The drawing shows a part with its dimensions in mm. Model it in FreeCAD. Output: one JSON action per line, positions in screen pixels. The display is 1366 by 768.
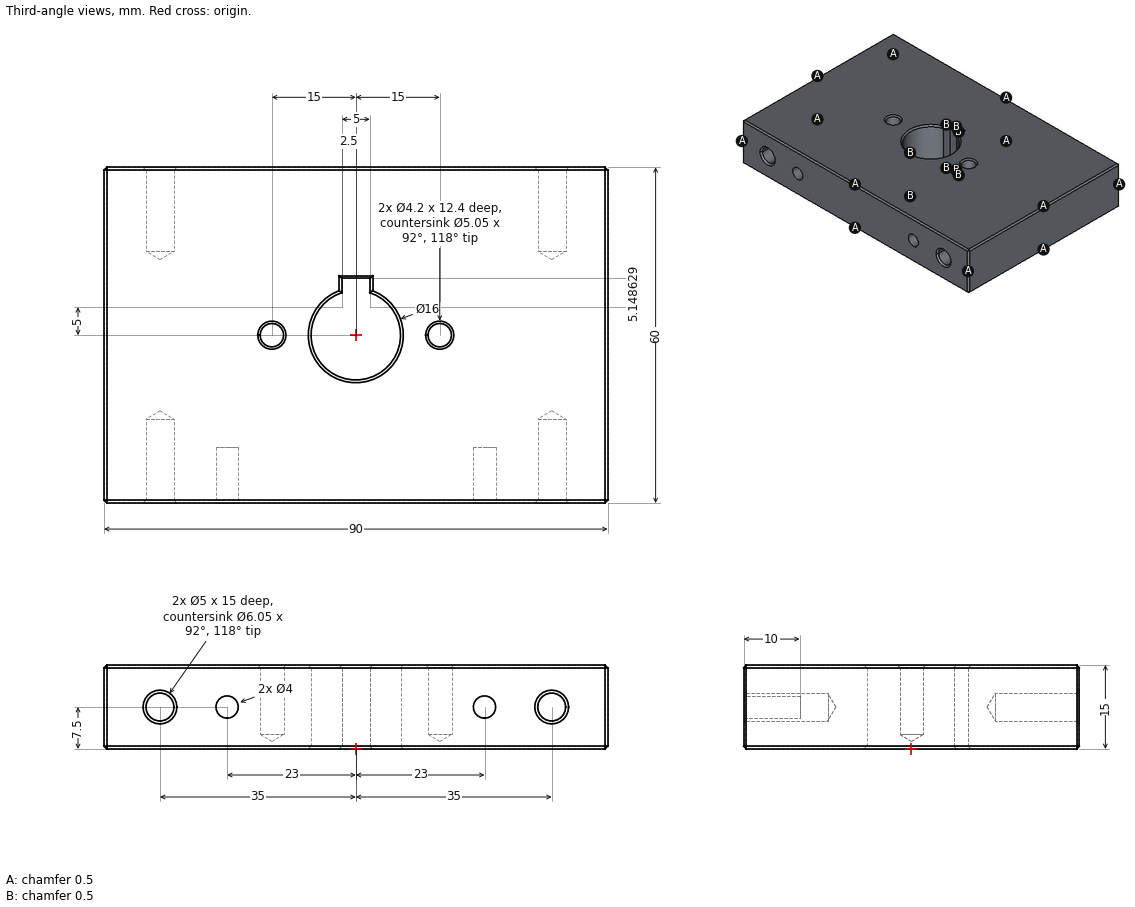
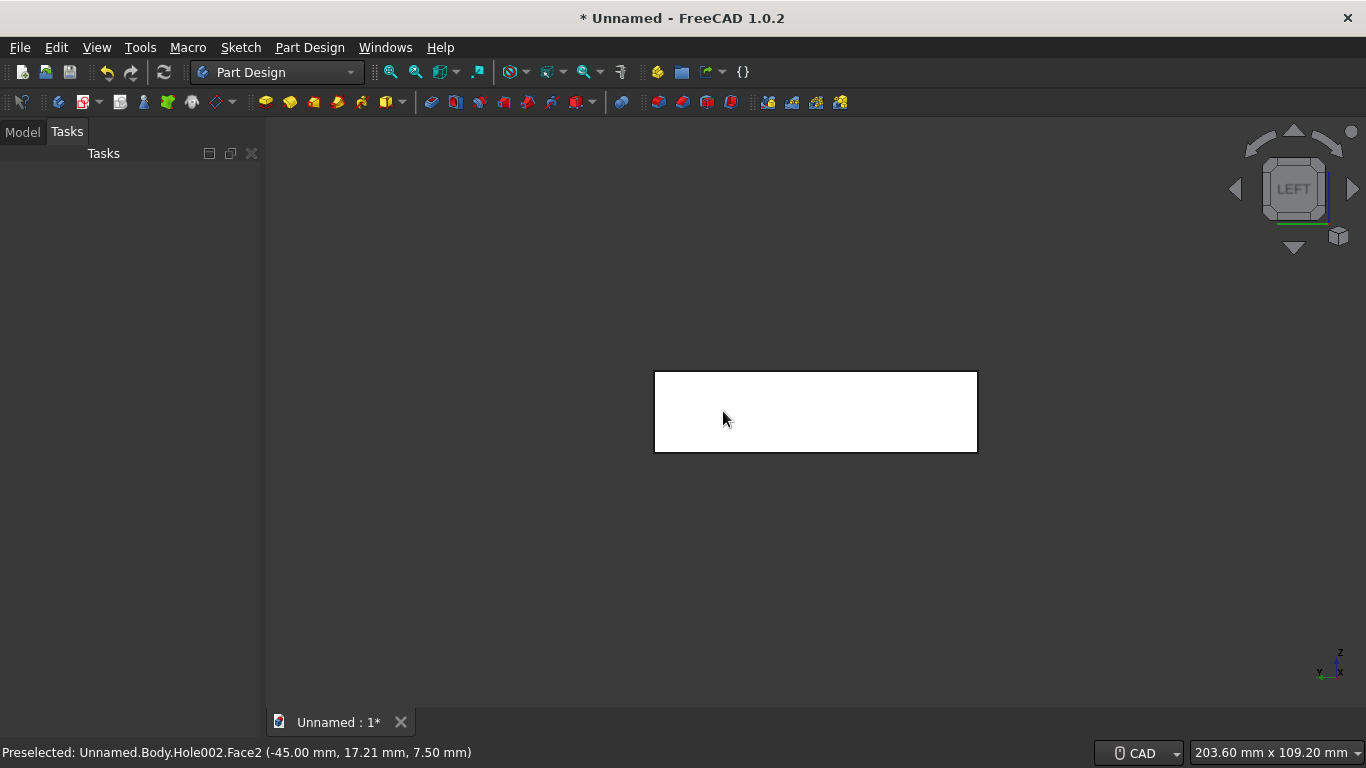
{"action": "left_click", "coordinate": [684, 102]}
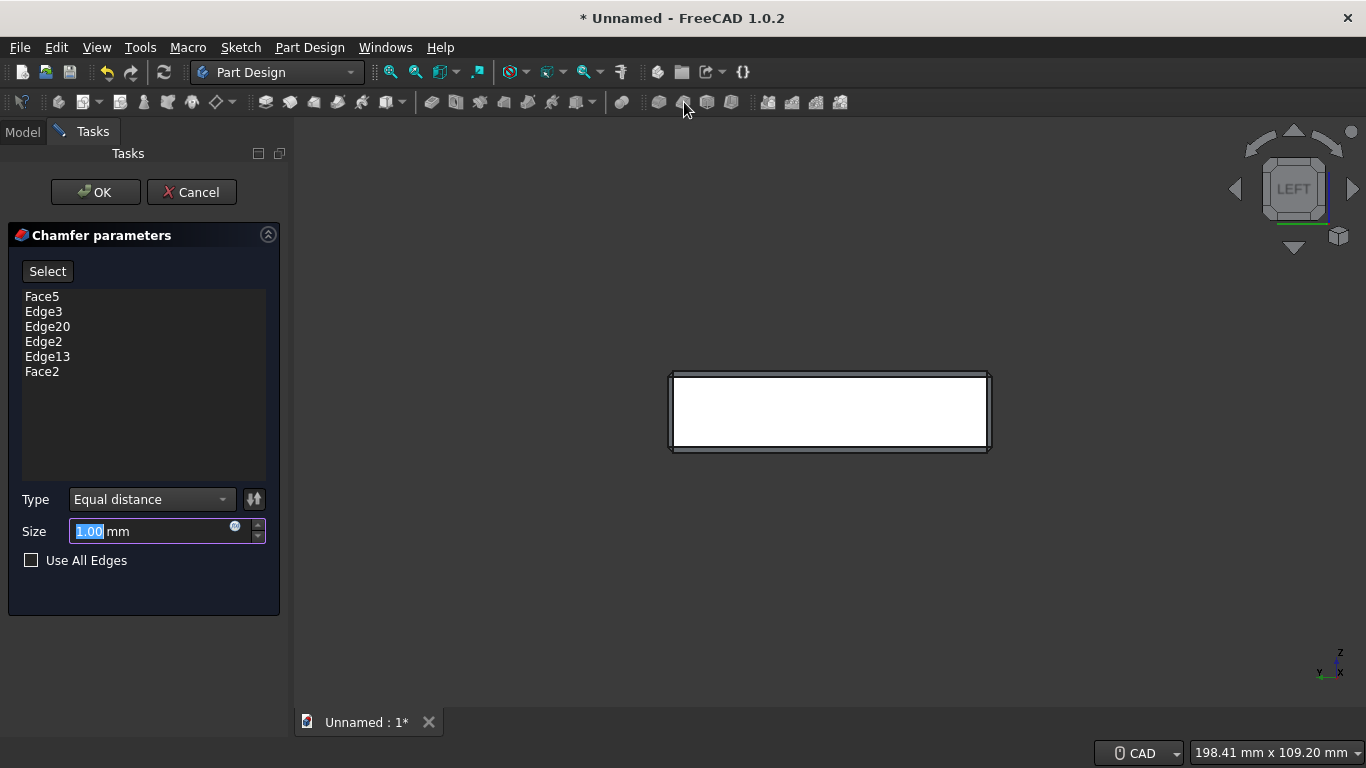
{"action": "type", "text": "0.5"}
{"action": "key", "text": "Tab"}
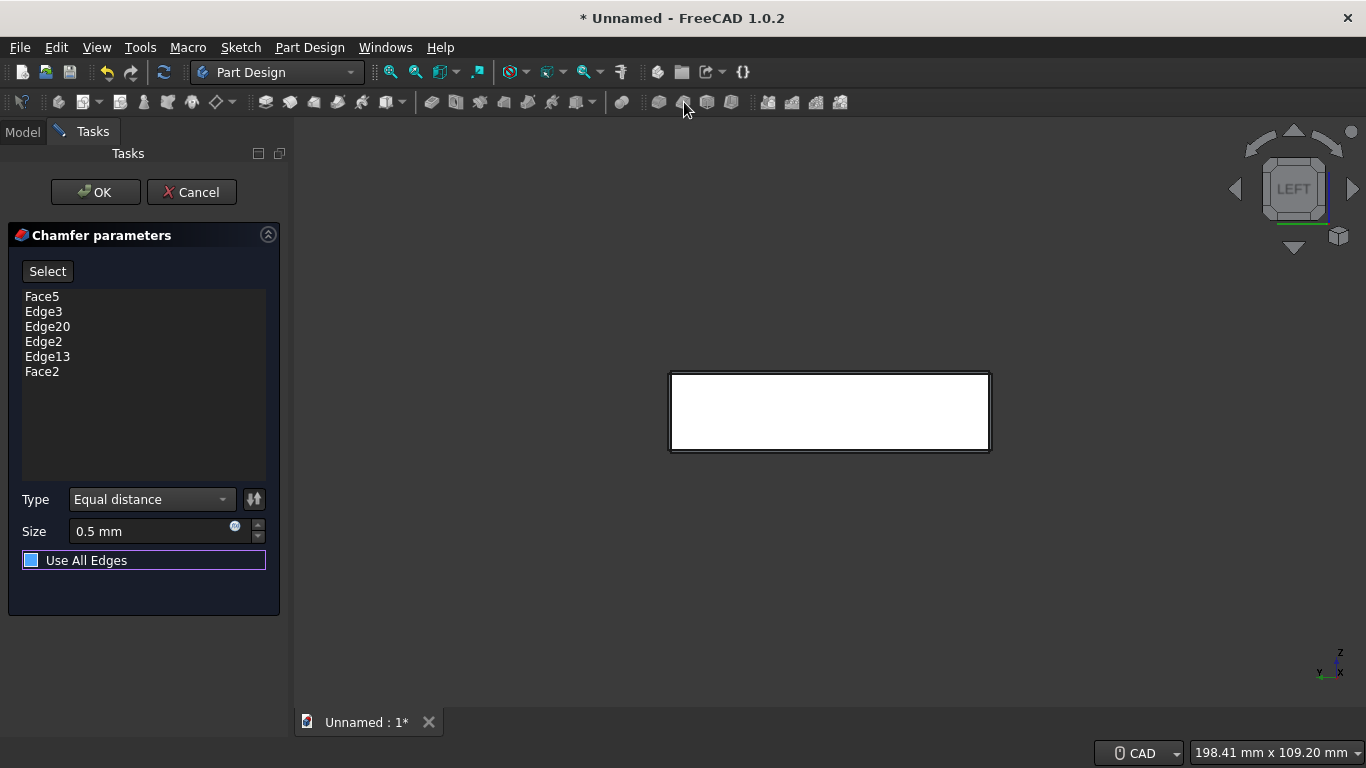
{"action": "left_click", "coordinate": [96, 192]}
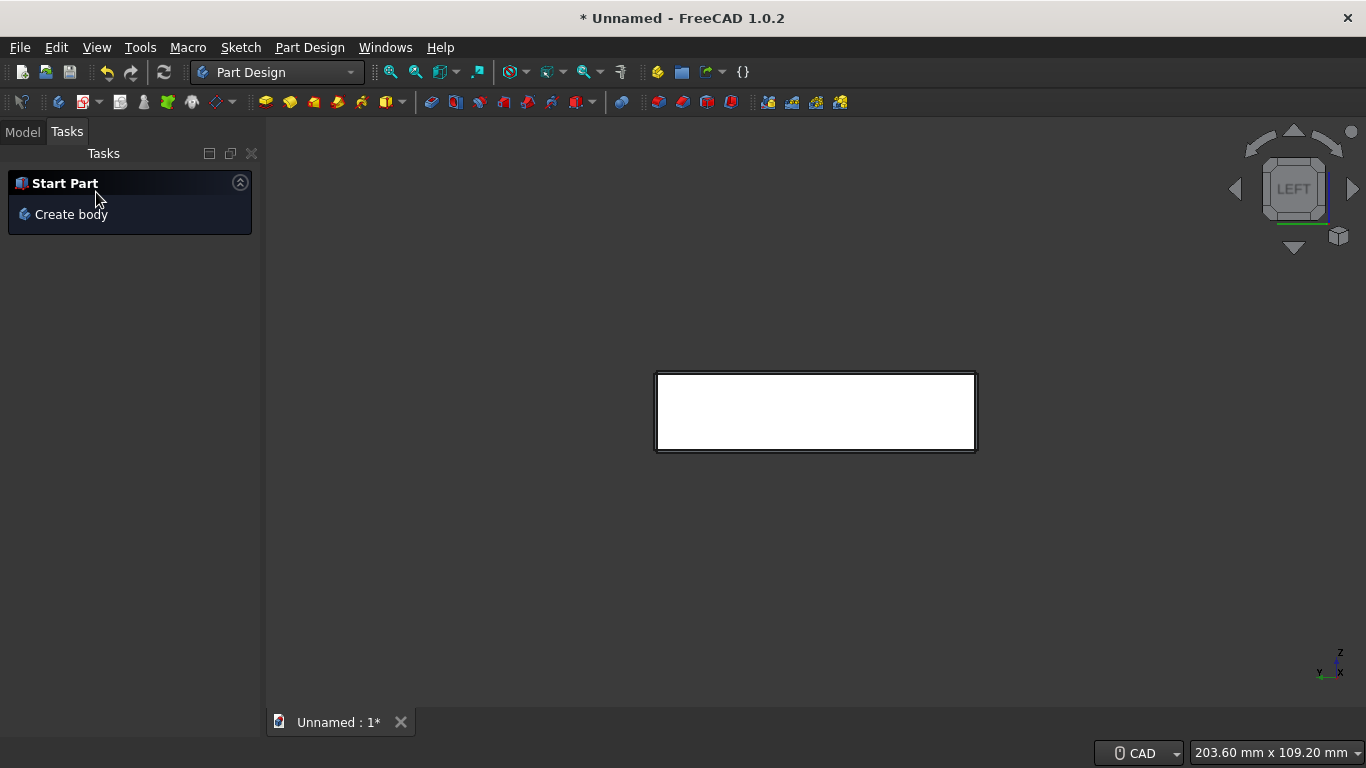
{"action": "key", "text": "v f"}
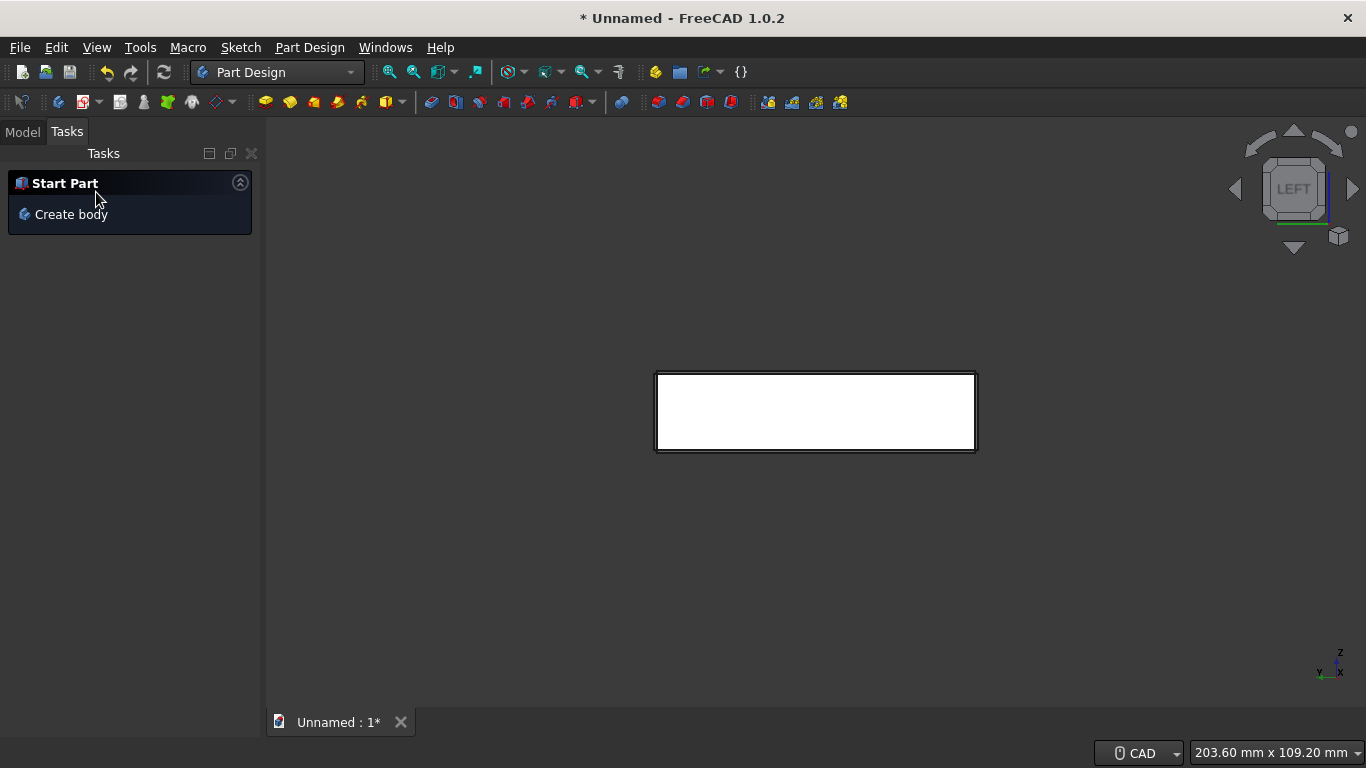
{"action": "key", "text": "0"}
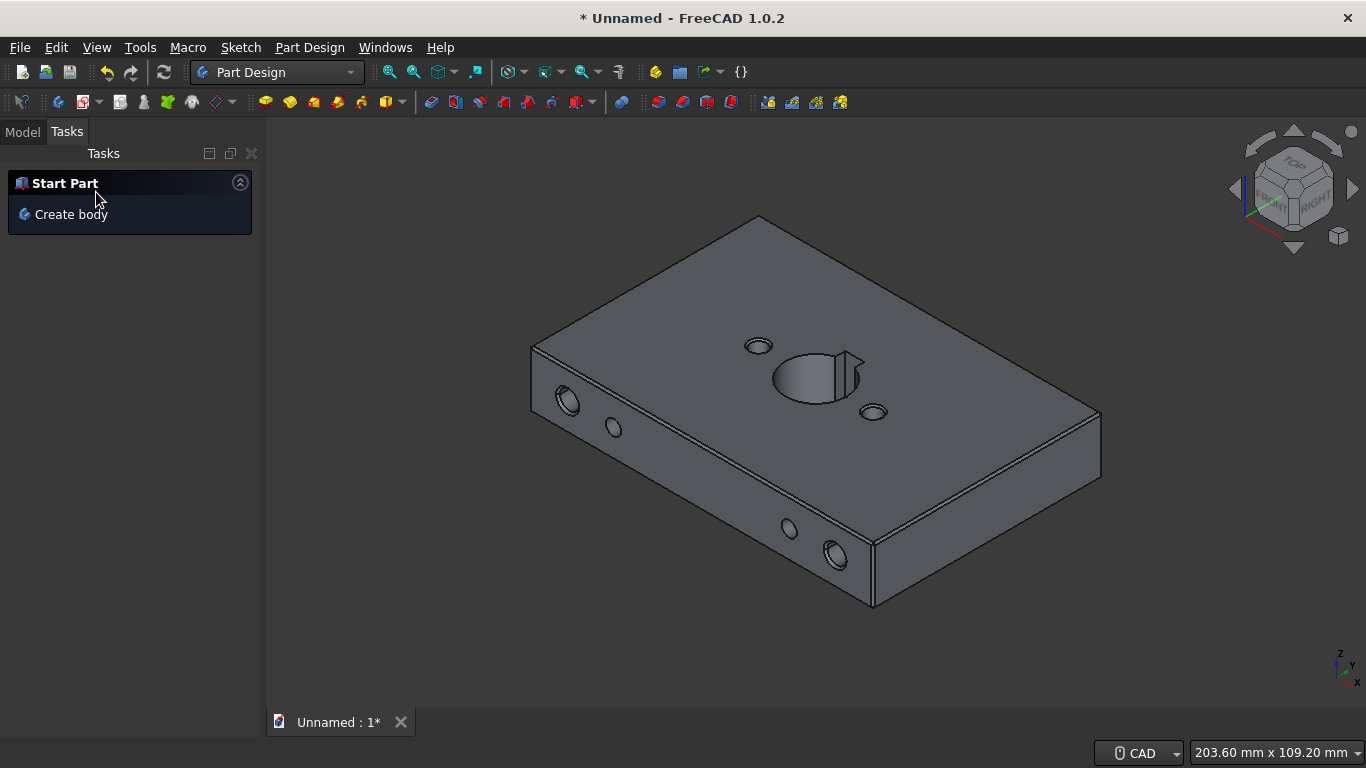
{"action": "left_click", "coordinate": [774, 371]}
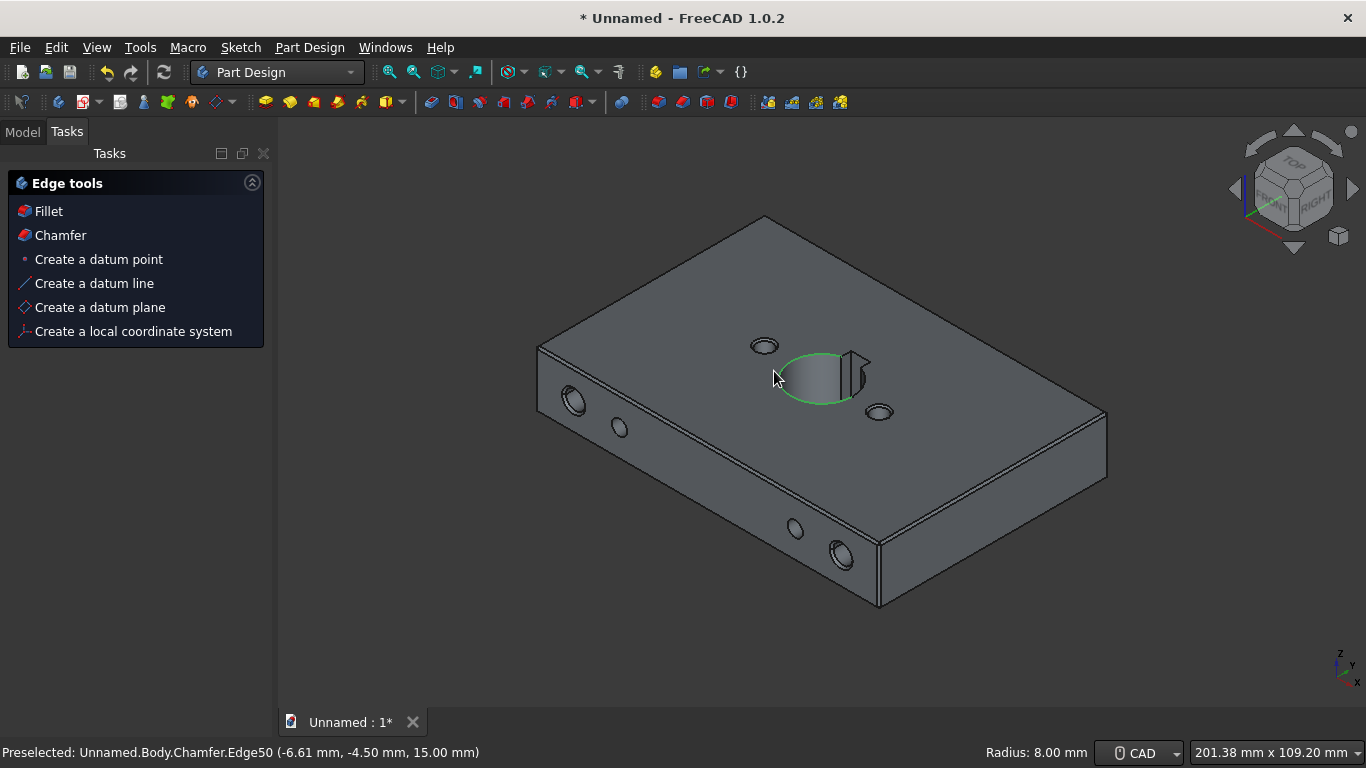
{"action": "left_click", "coordinate": [847, 352], "text": "ctrl"}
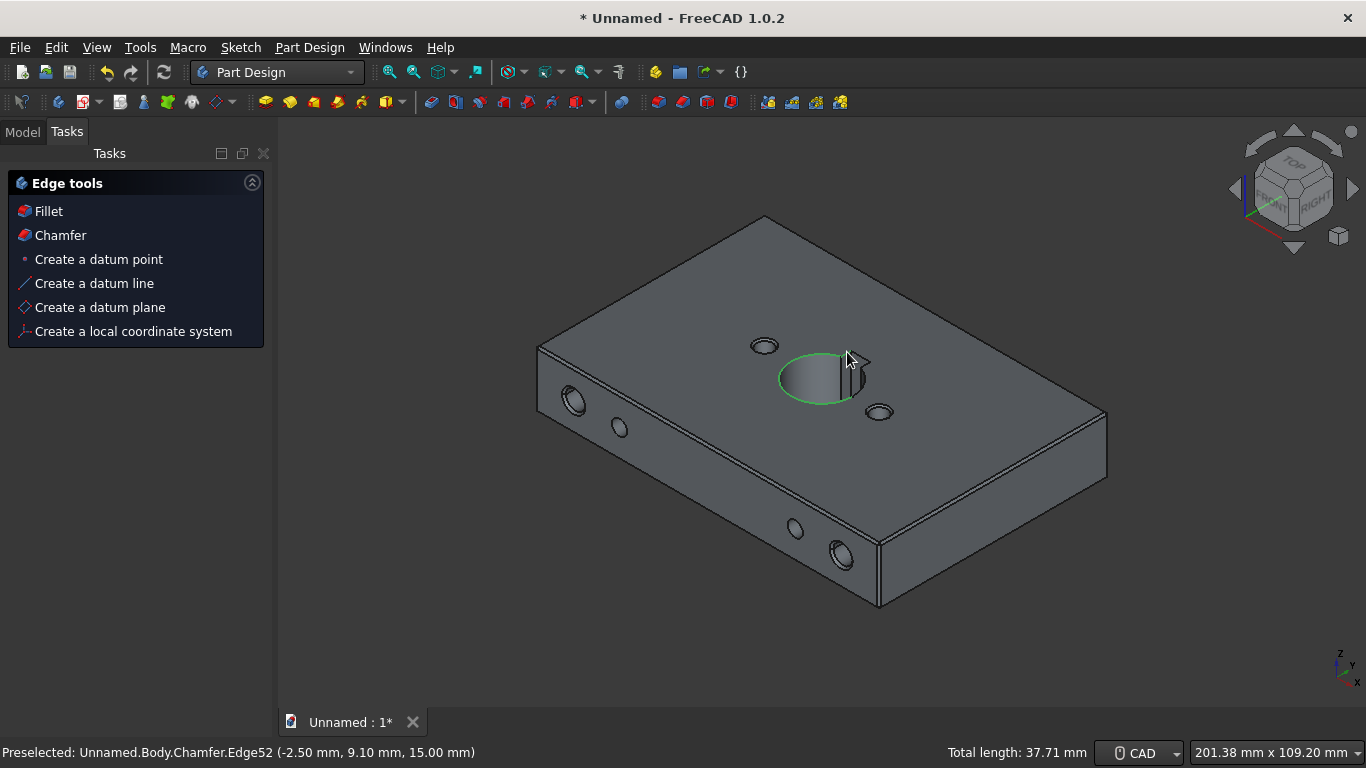
{"action": "left_click", "coordinate": [861, 356], "text": "ctrl"}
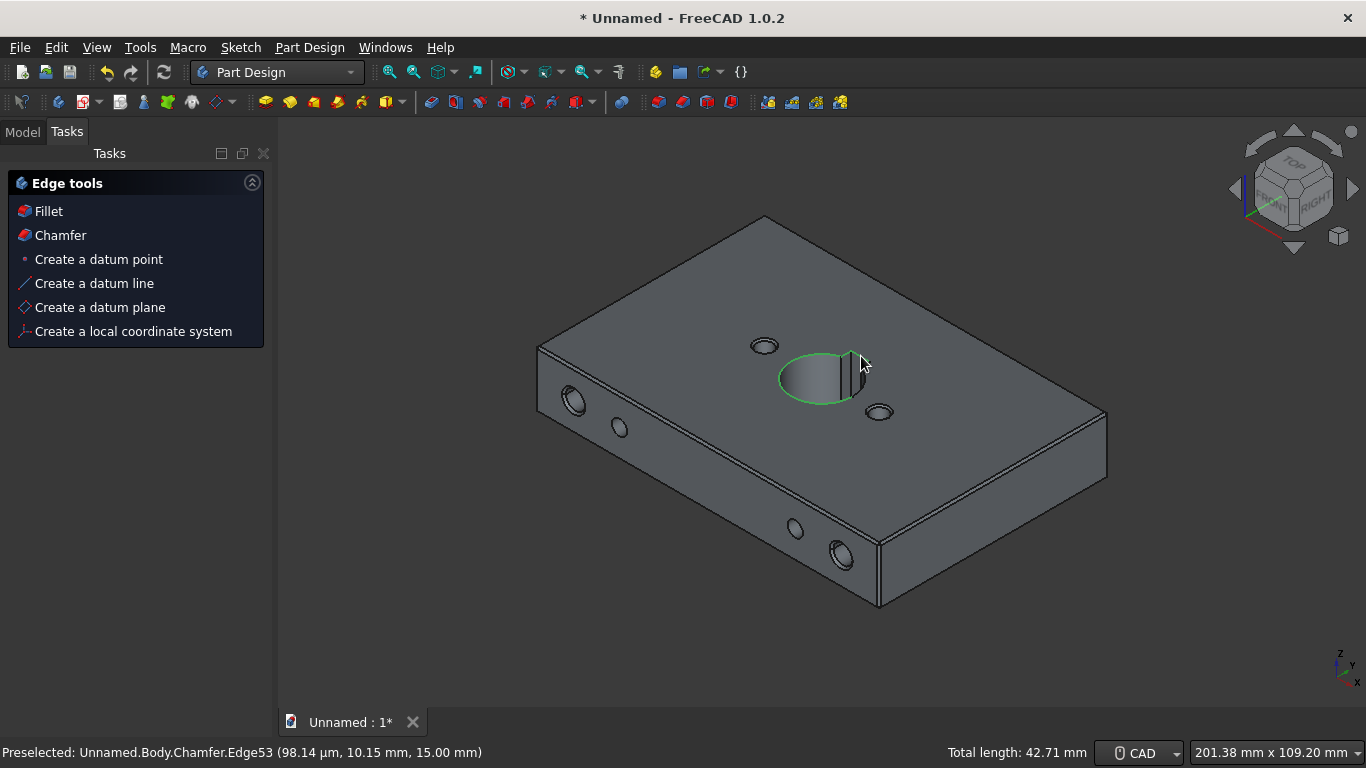
{"action": "key", "text": "2"}